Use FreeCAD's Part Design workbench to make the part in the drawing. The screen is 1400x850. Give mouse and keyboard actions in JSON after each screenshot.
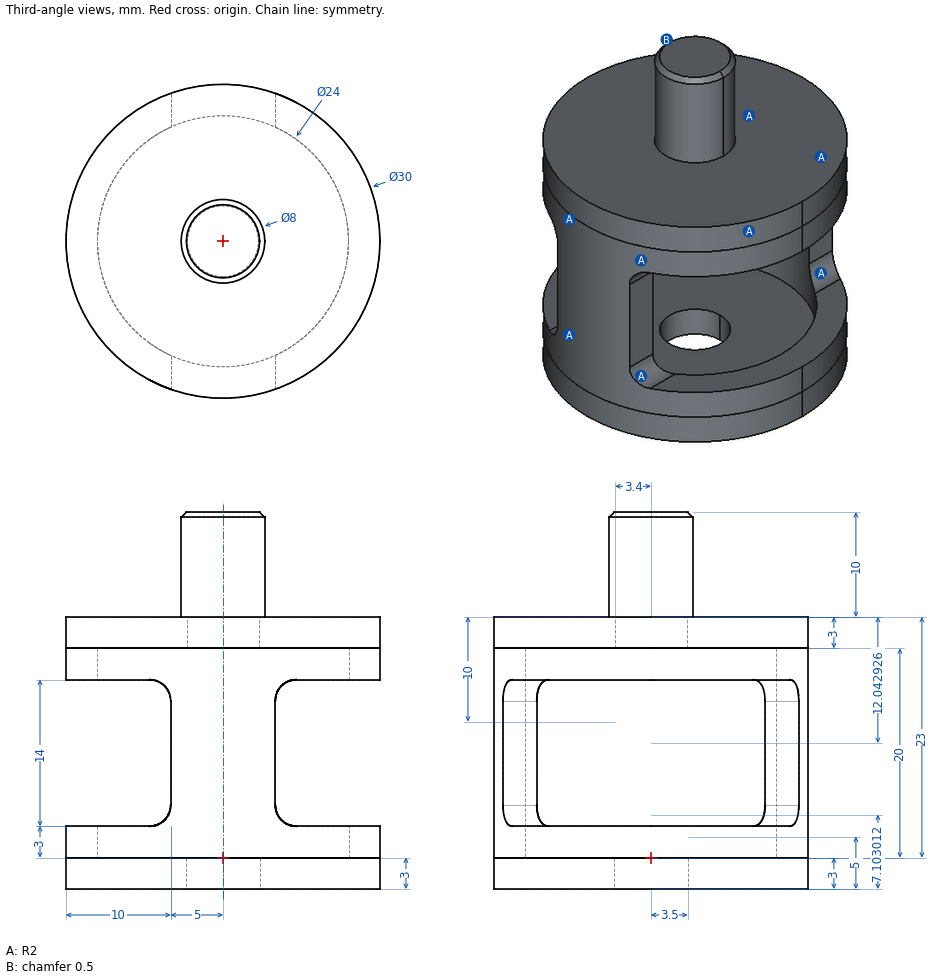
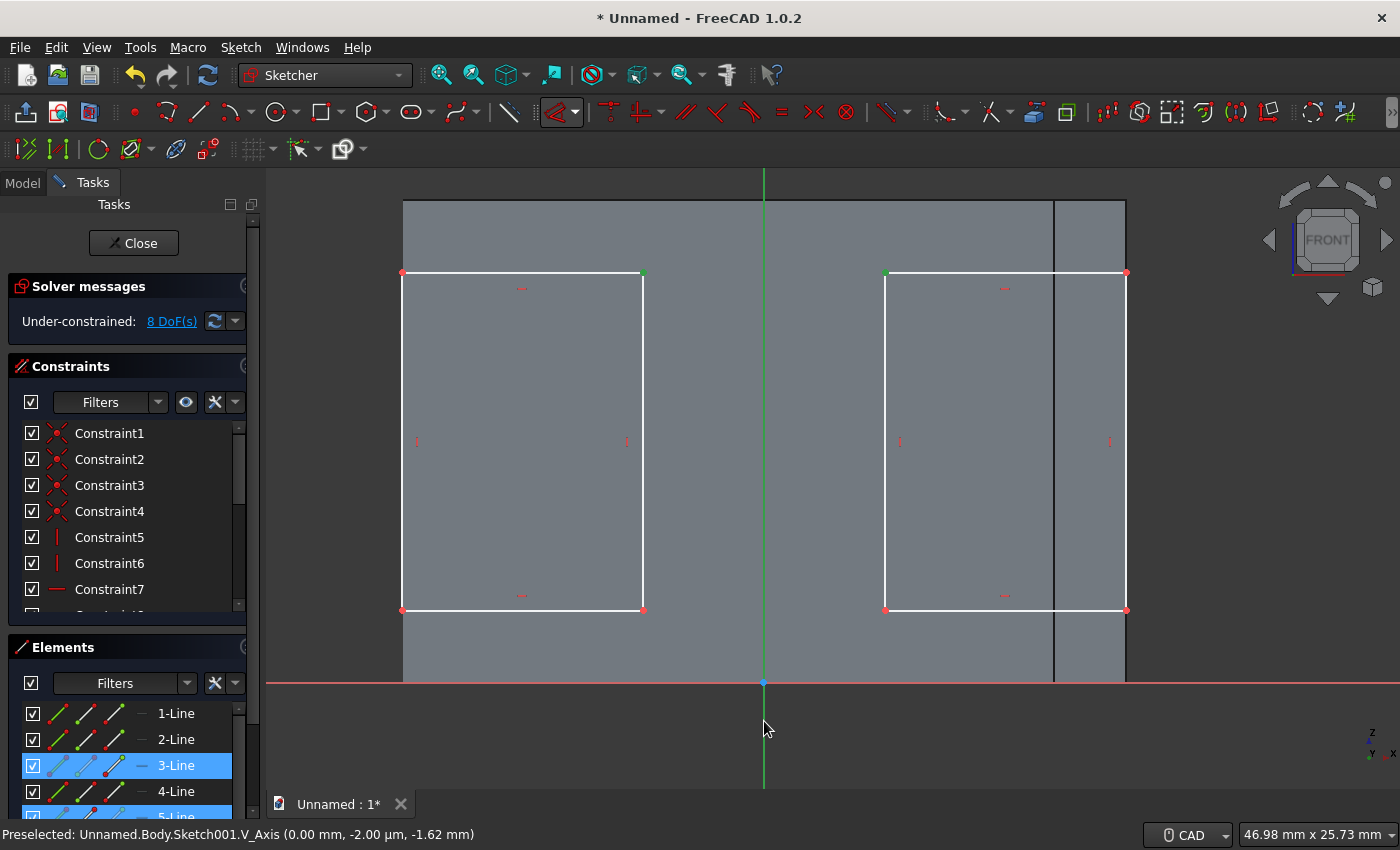
{"action": "left_click", "coordinate": [814, 112]}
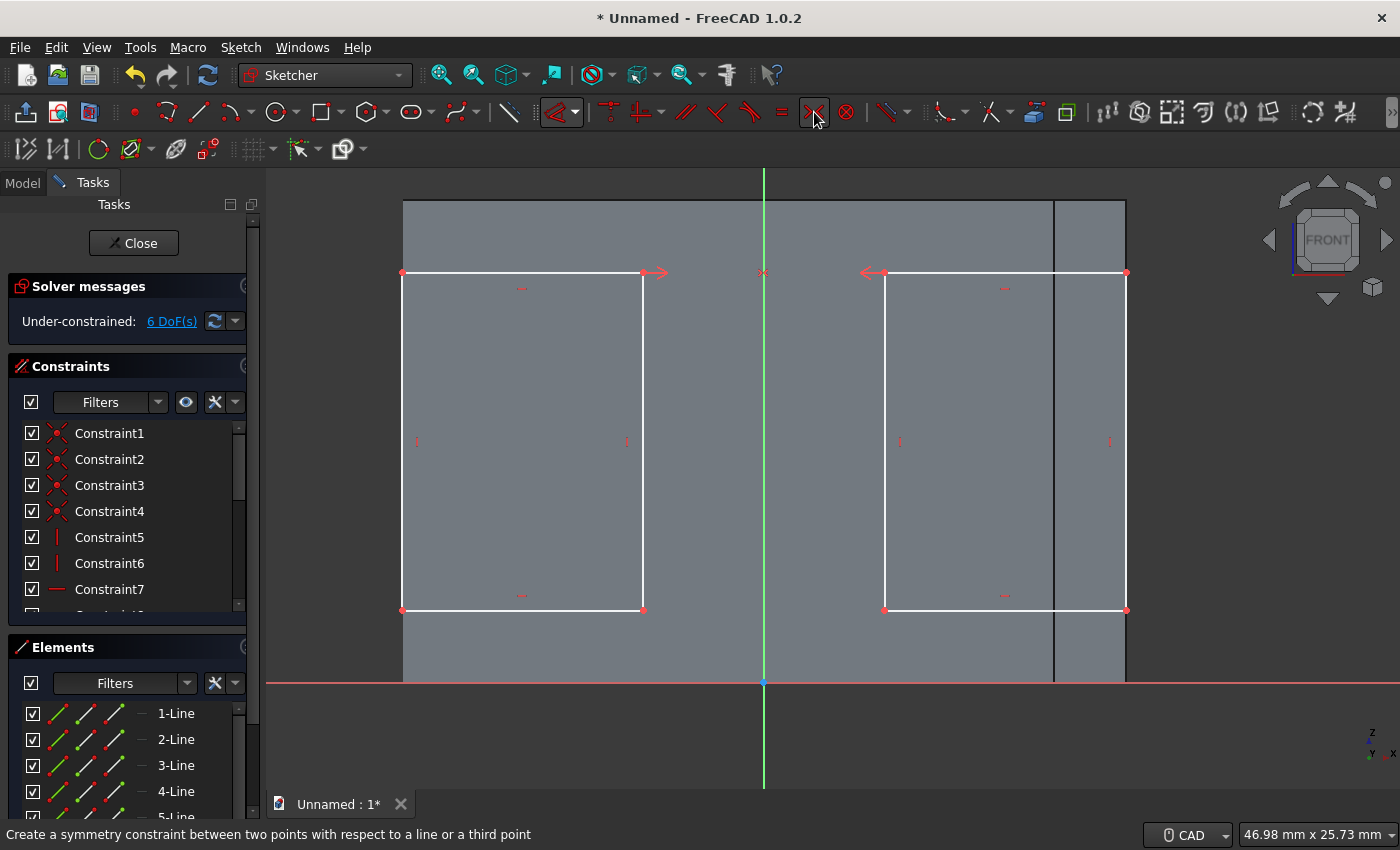
{"action": "left_click", "coordinate": [402, 611]}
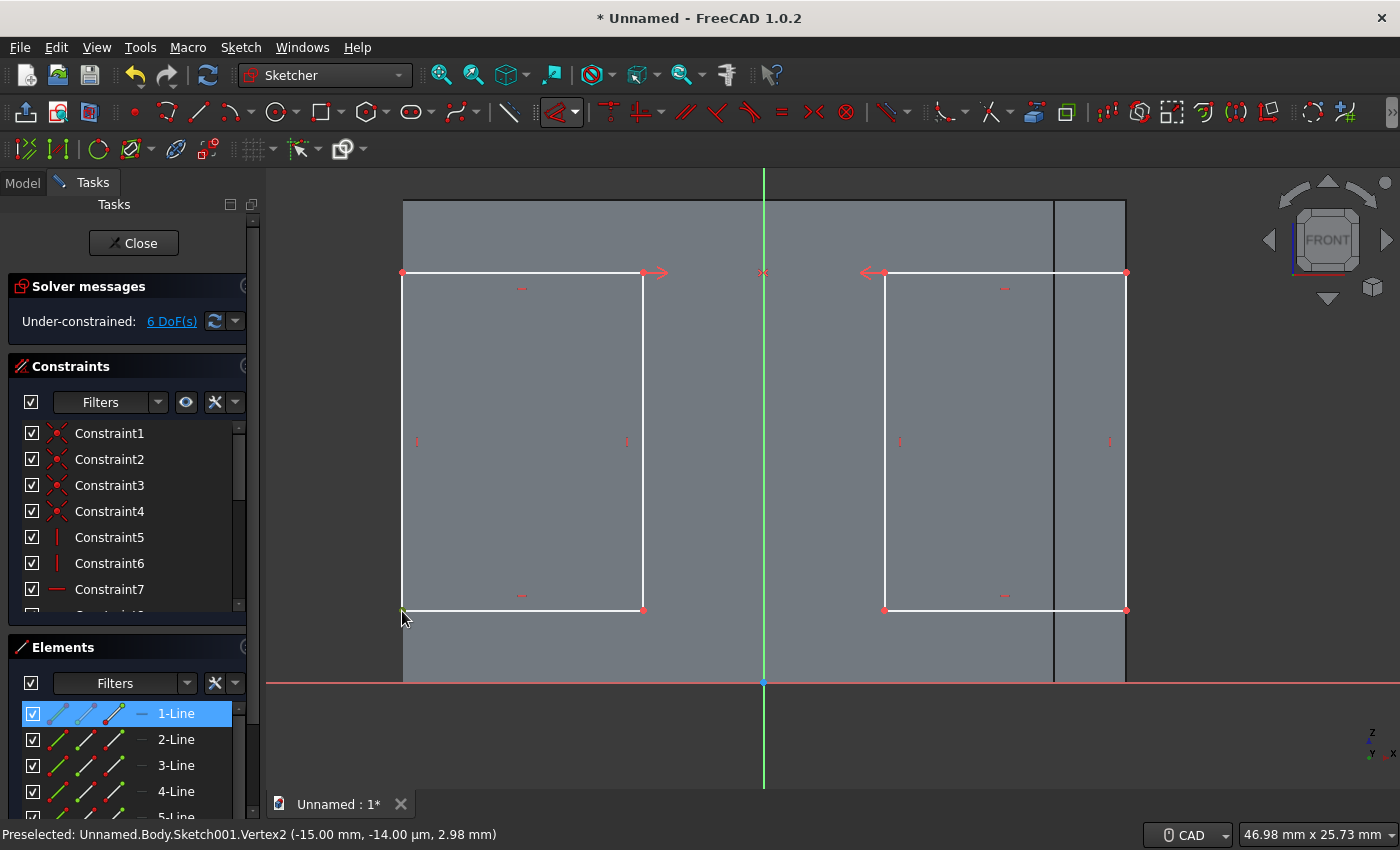
{"action": "left_click", "coordinate": [1126, 611]}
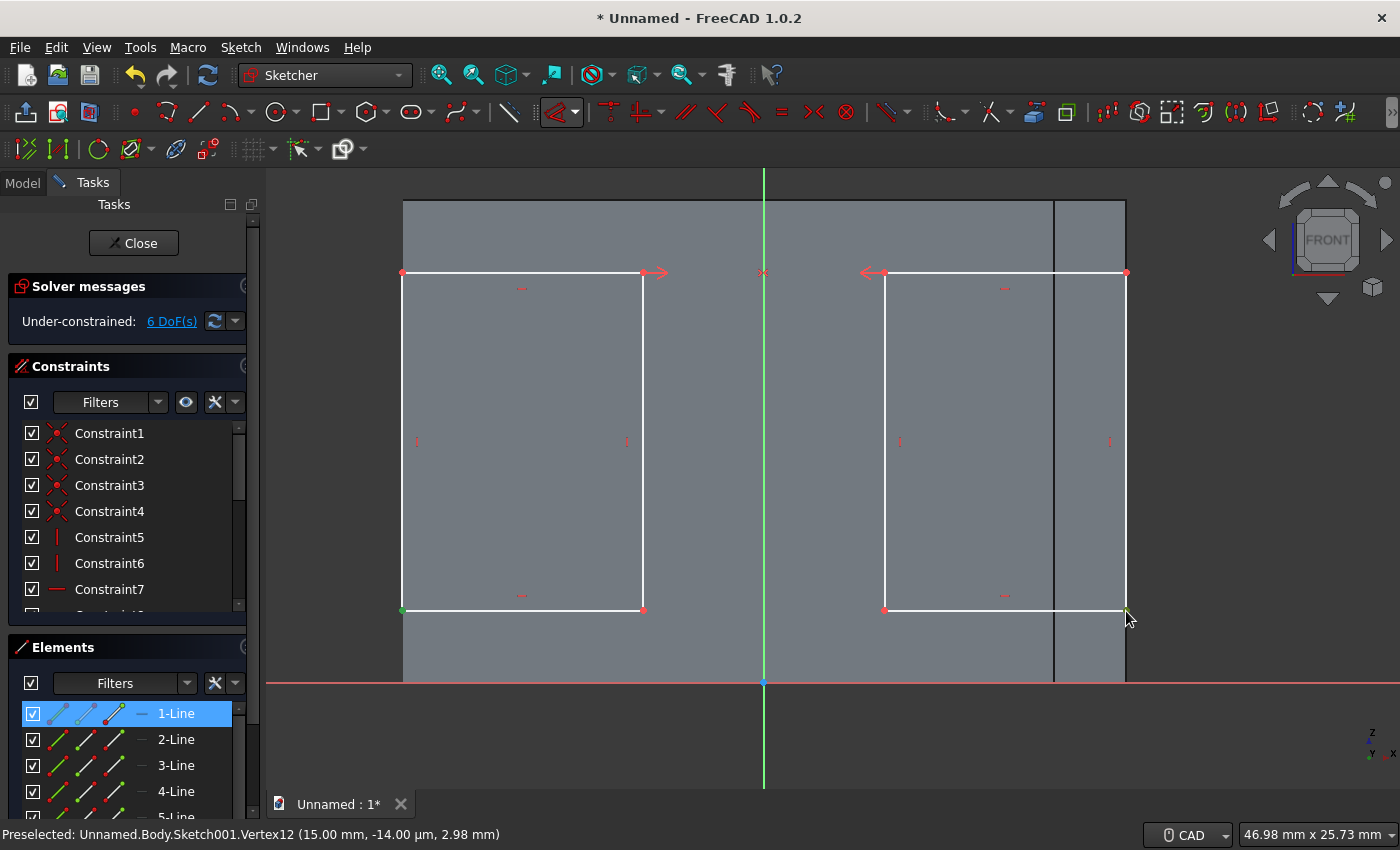
{"action": "left_click", "coordinate": [764, 721]}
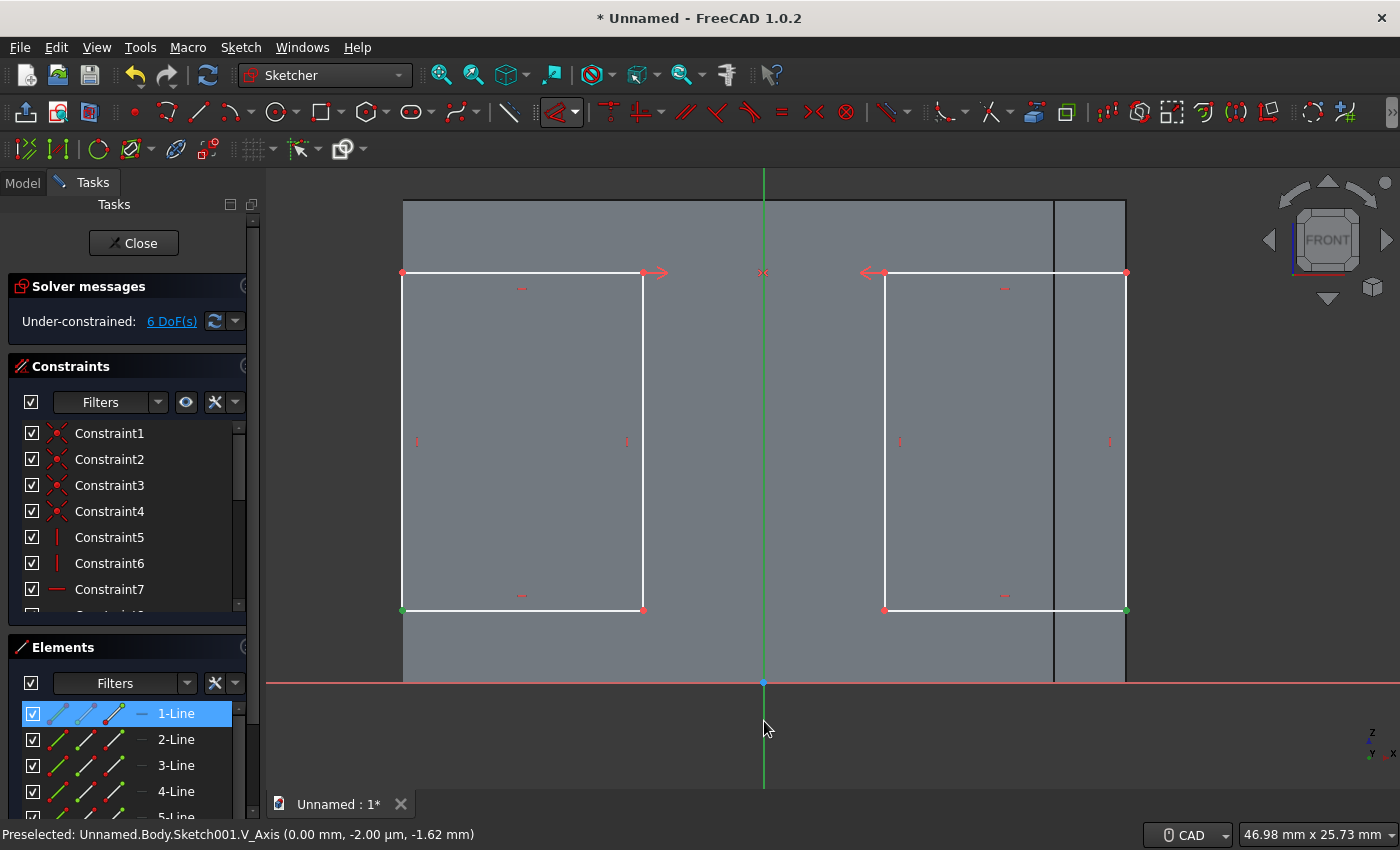
{"action": "key", "text": "s"}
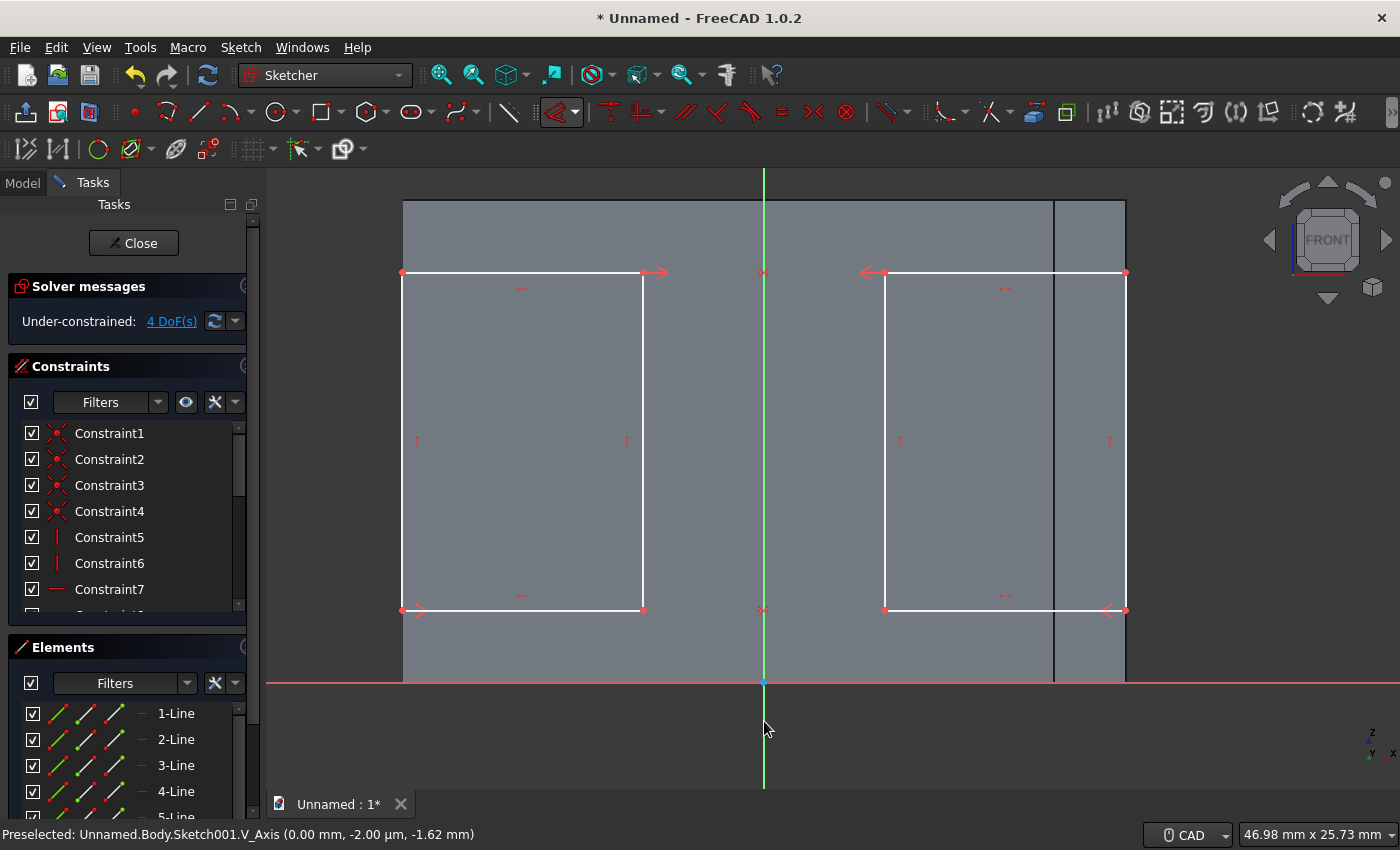
{"action": "left_click", "coordinate": [402, 374]}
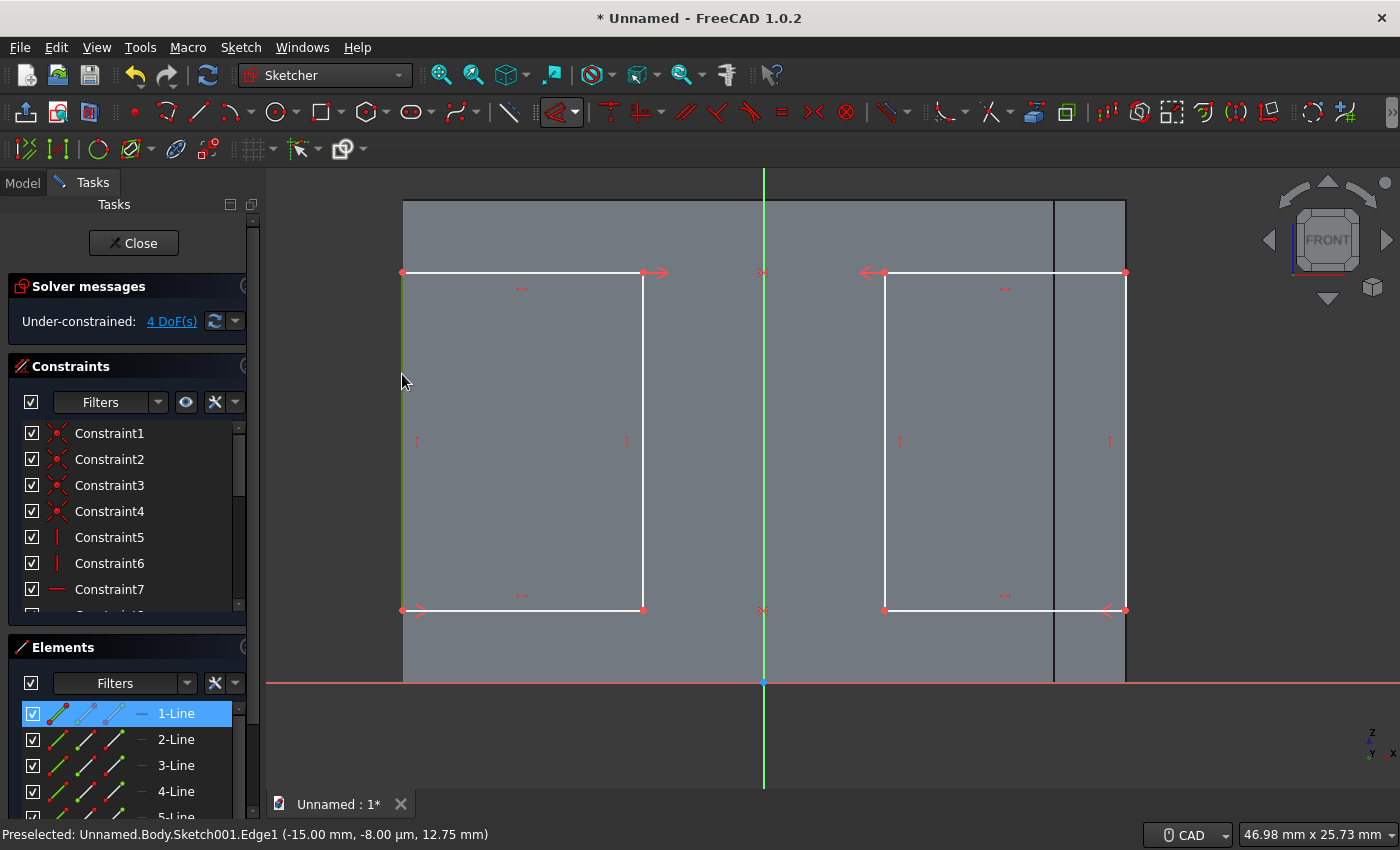
{"action": "key", "text": "i"}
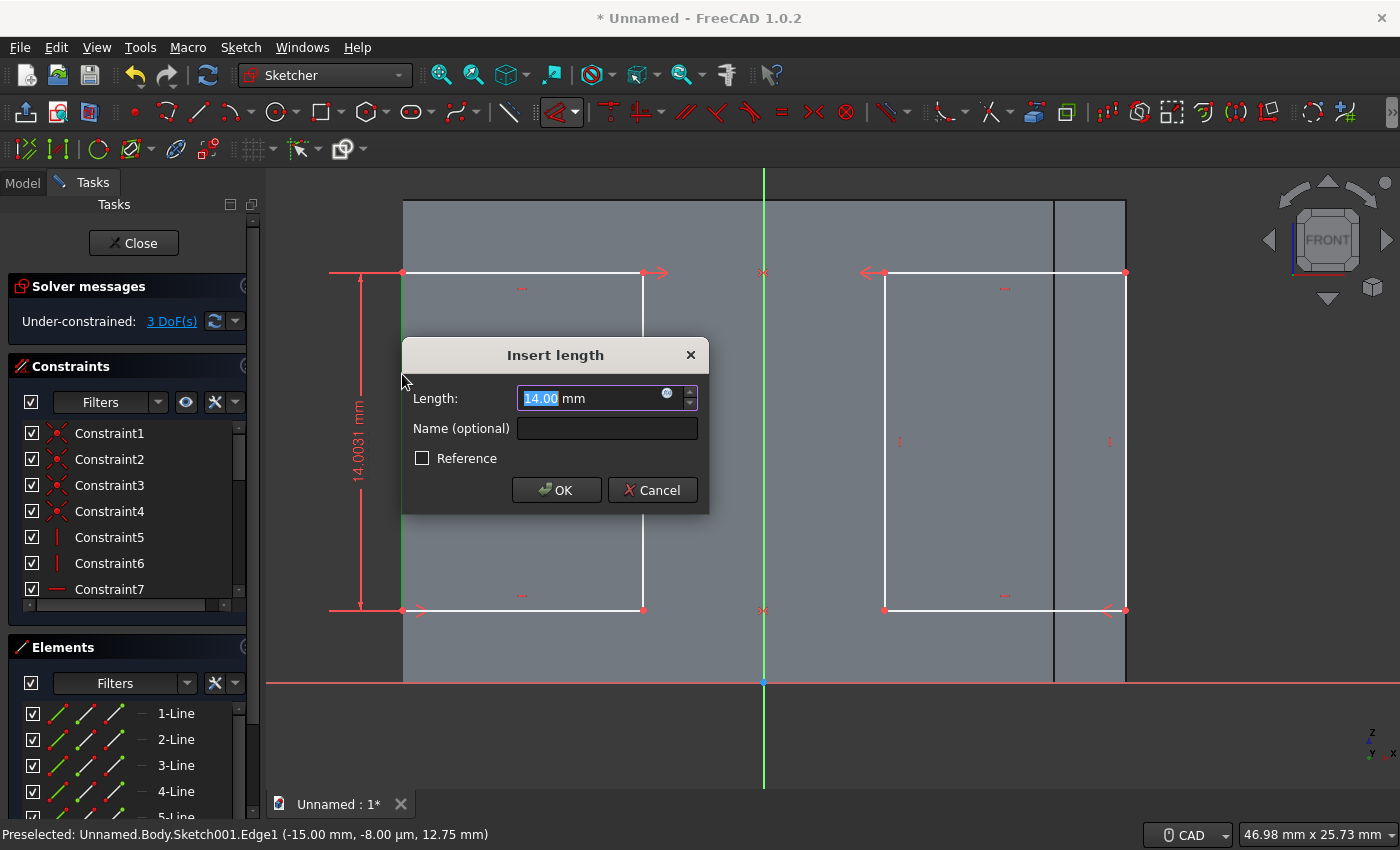
{"action": "type", "text": "14"}
{"action": "key", "text": "Return"}